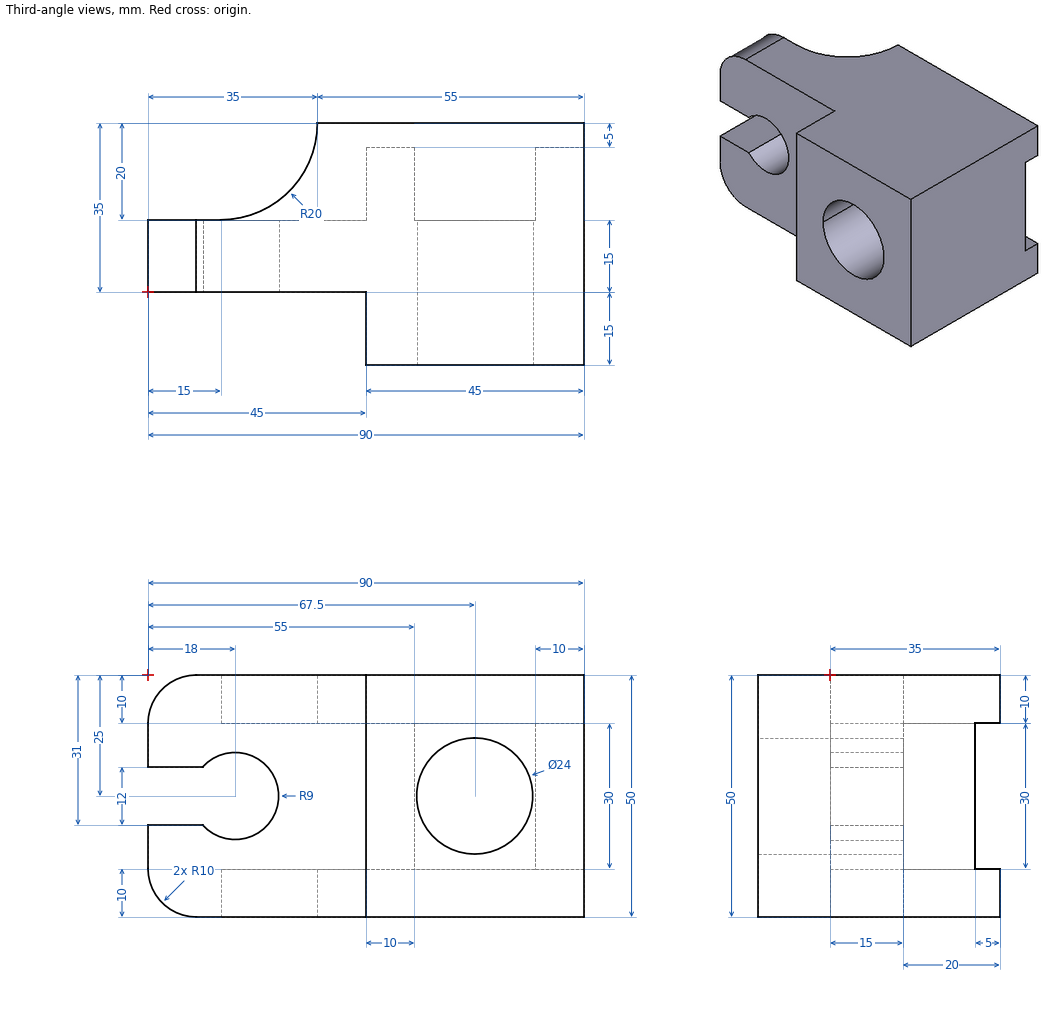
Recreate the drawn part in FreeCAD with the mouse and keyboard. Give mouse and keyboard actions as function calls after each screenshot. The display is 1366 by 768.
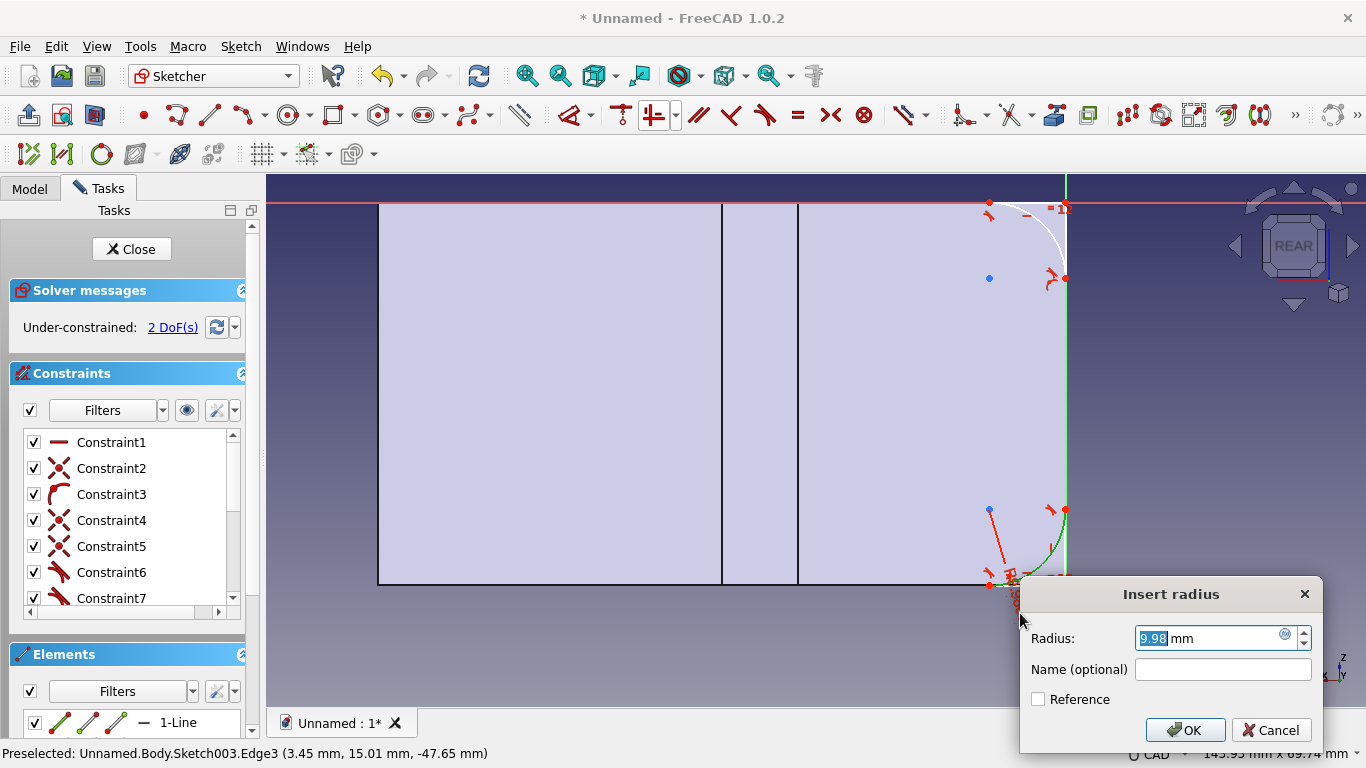
text(10)
key(Return)
key(Escape)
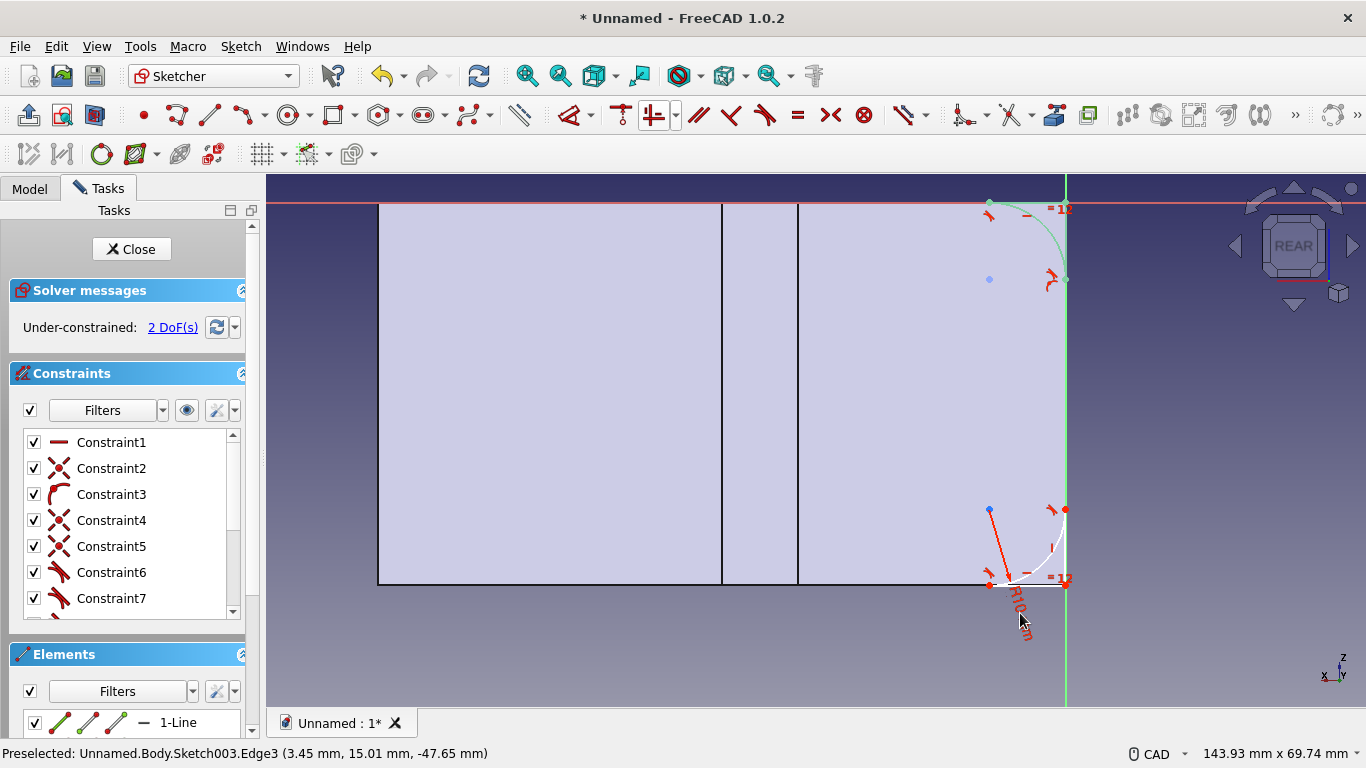
click(1065, 586)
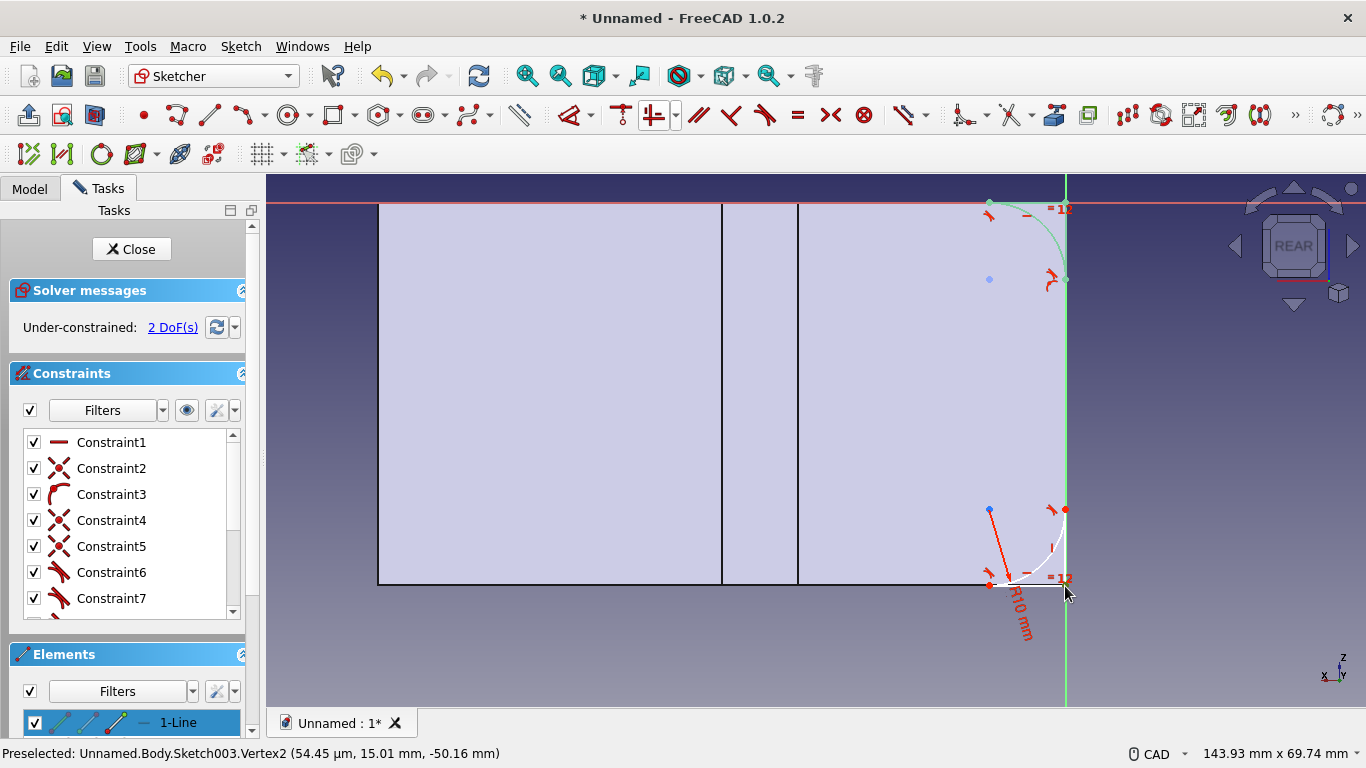
click(1066, 645)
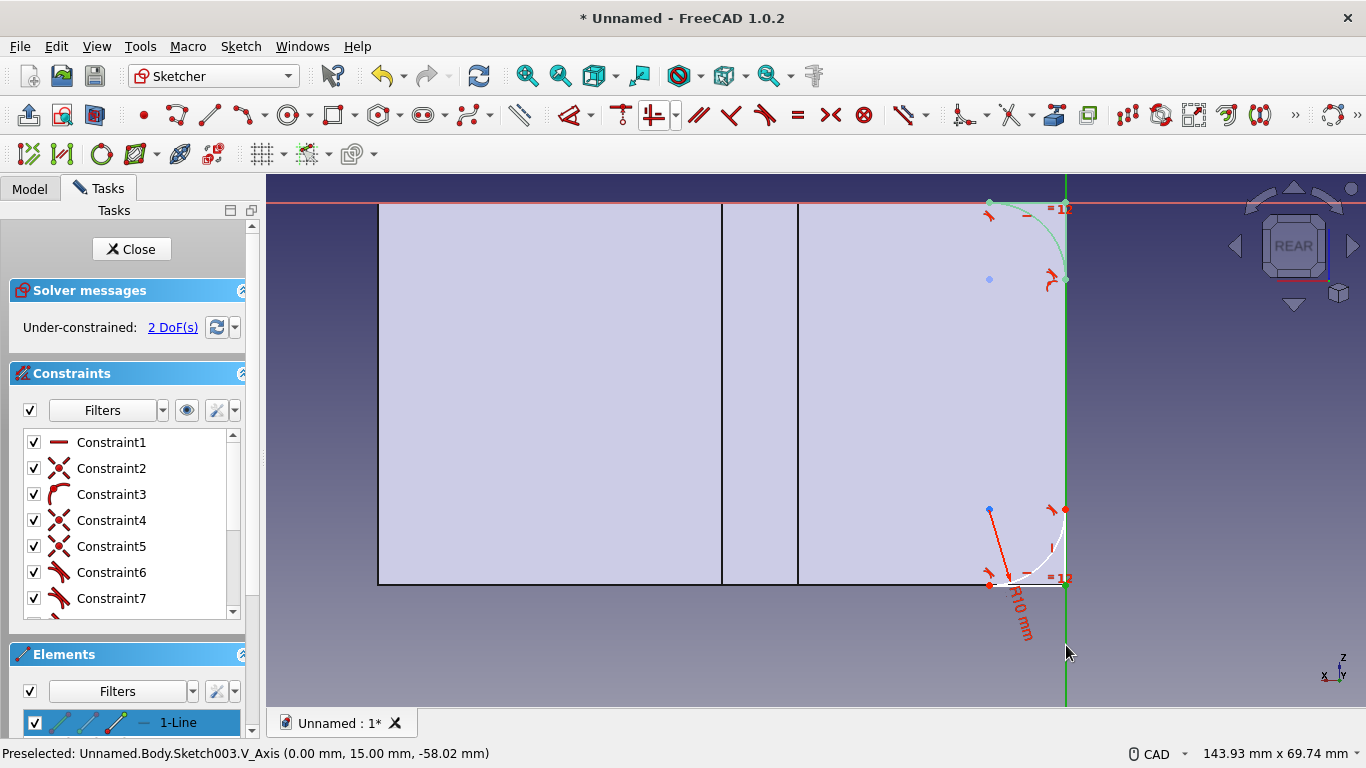
click(621, 116)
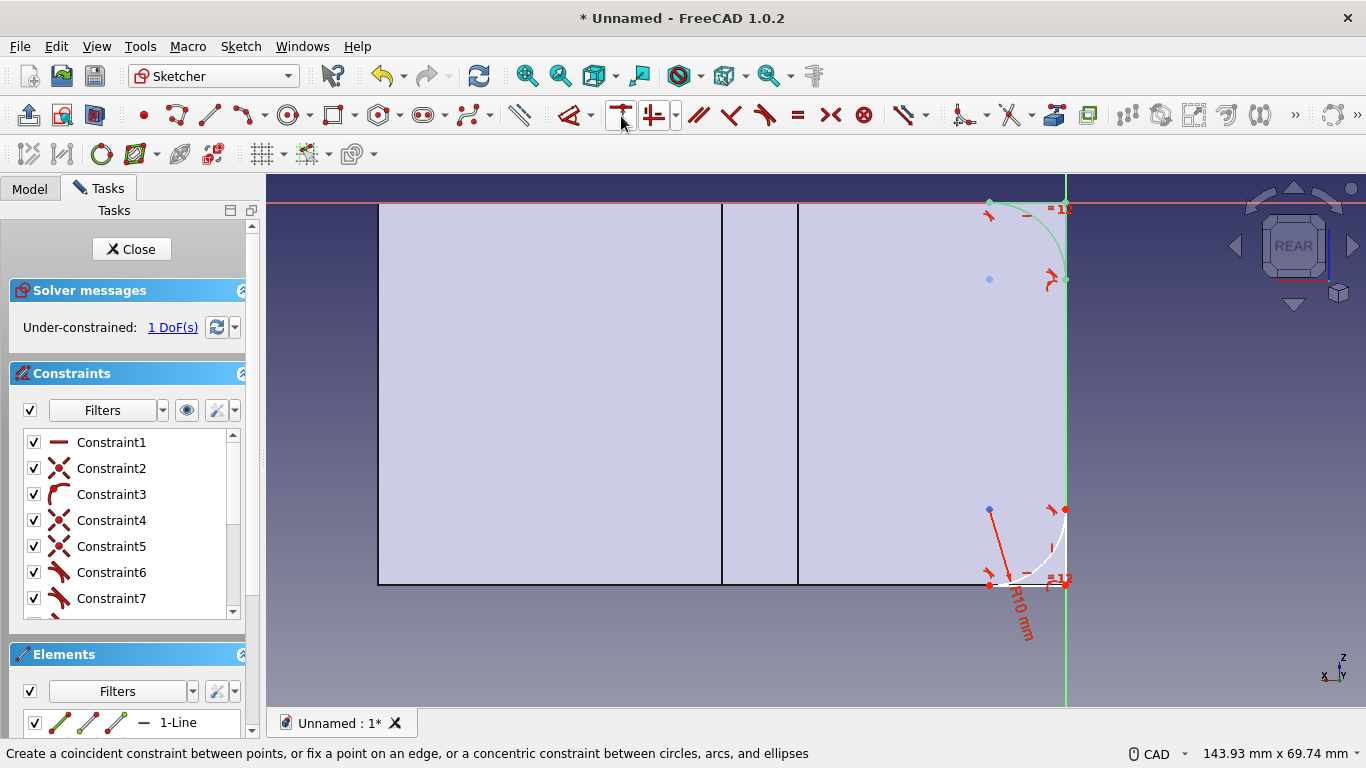
click(568, 116)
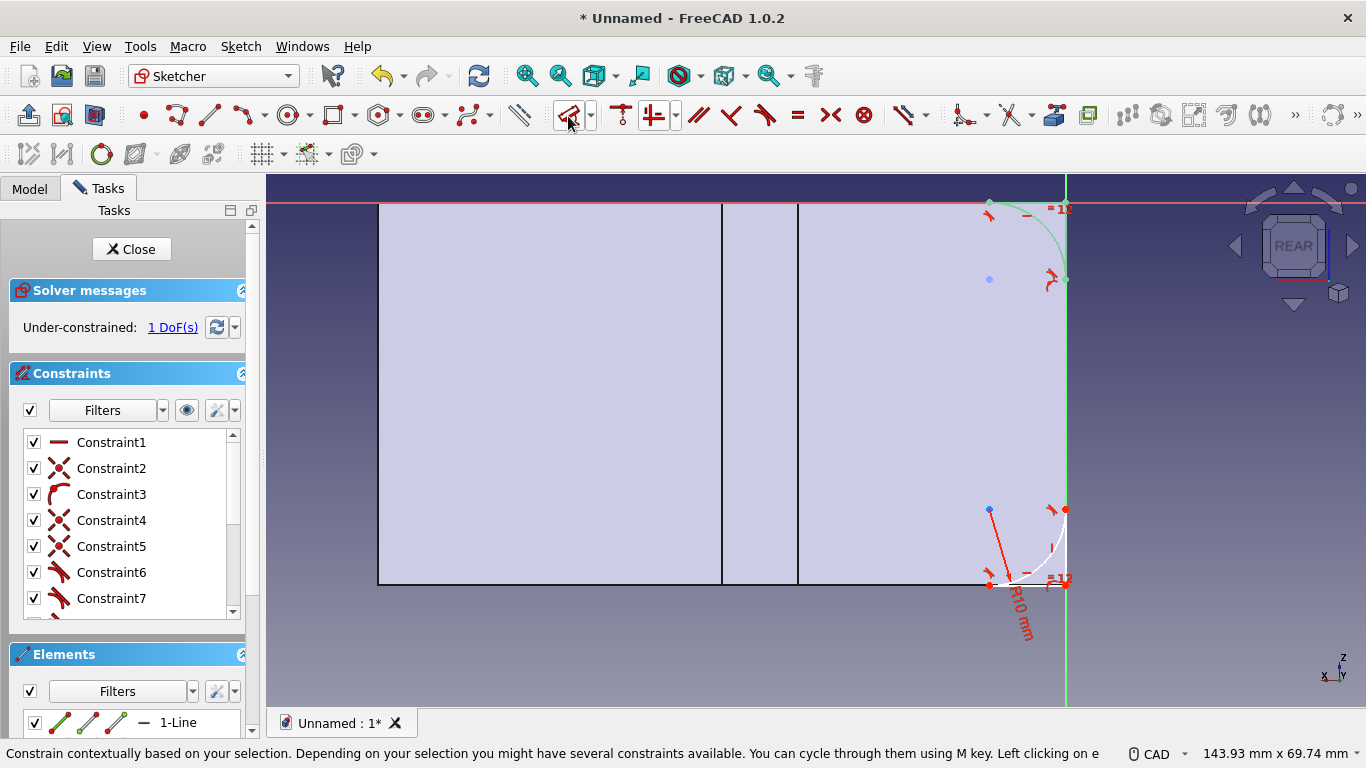
click(989, 586)
click(1100, 394)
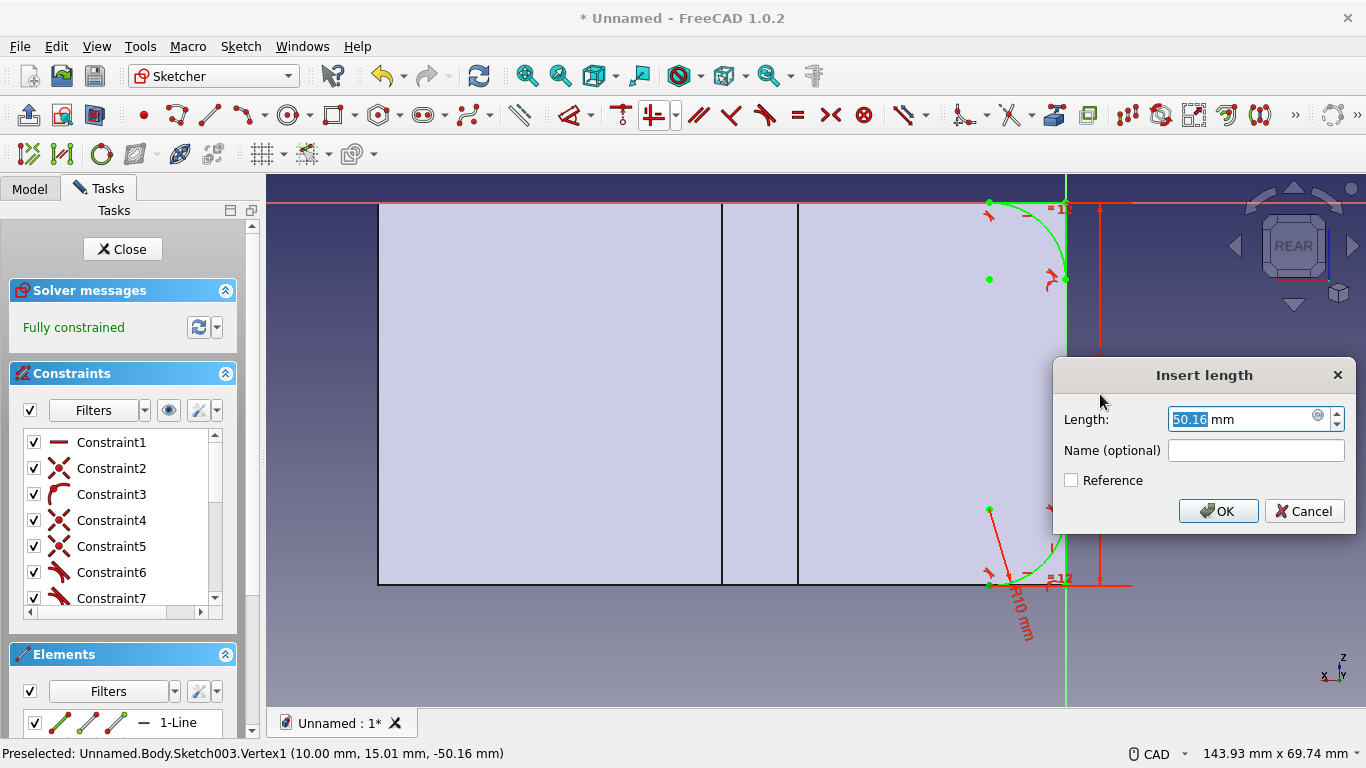
text(50)
key(Return)
key(Escape)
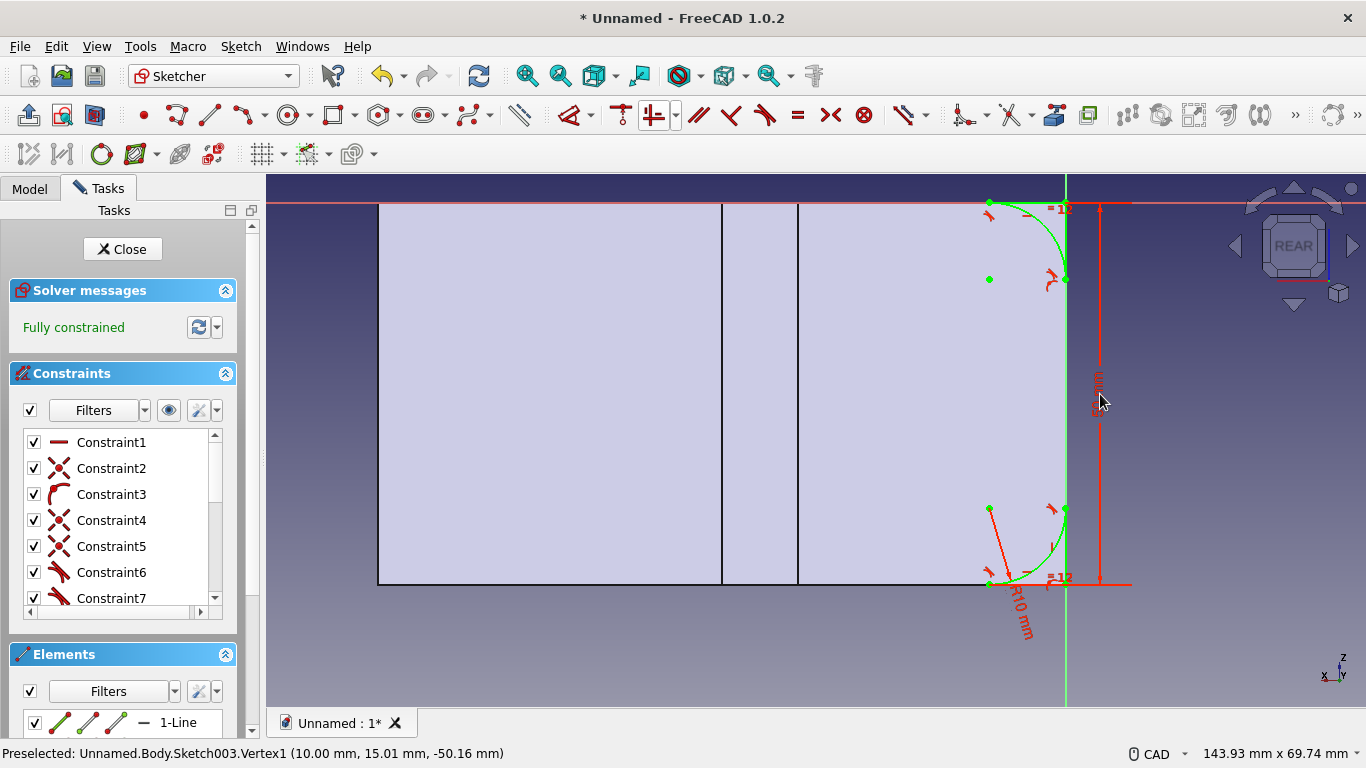
click(123, 249)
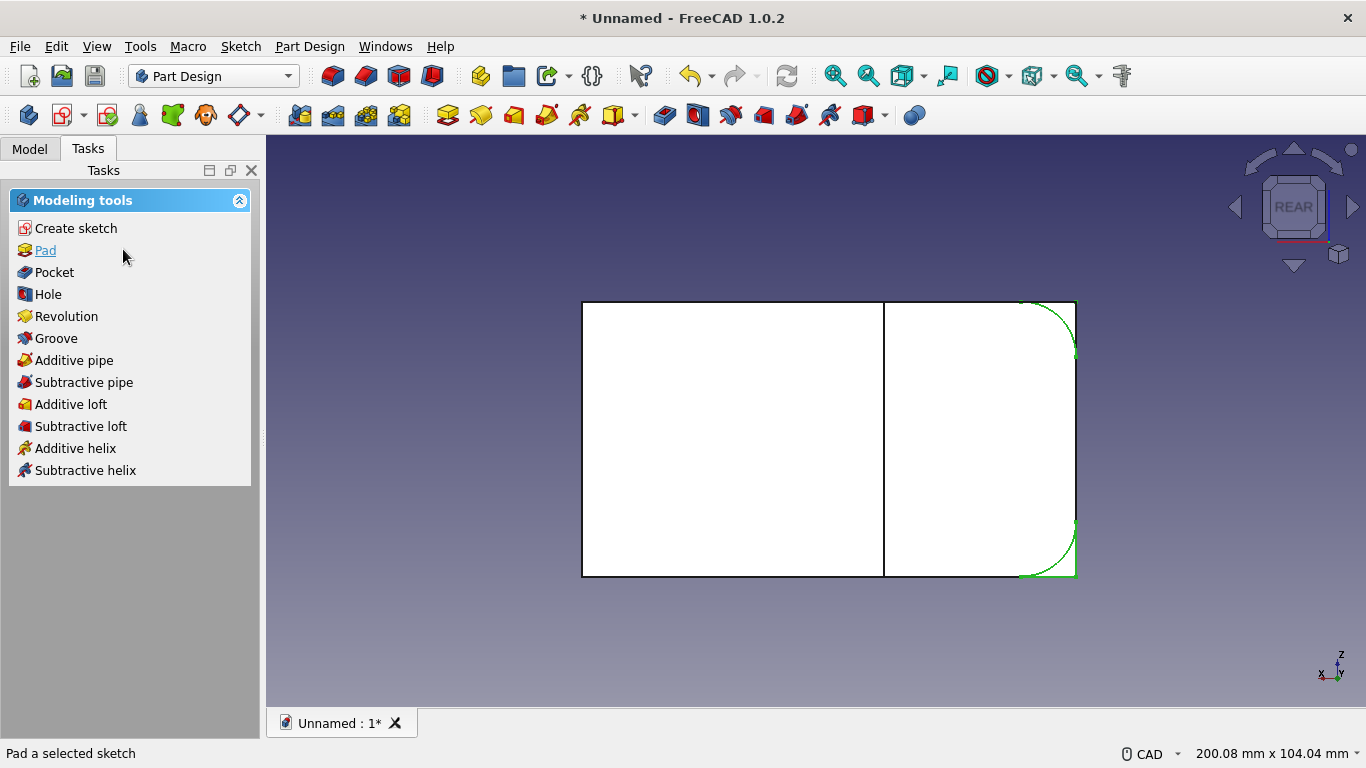
click(665, 116)